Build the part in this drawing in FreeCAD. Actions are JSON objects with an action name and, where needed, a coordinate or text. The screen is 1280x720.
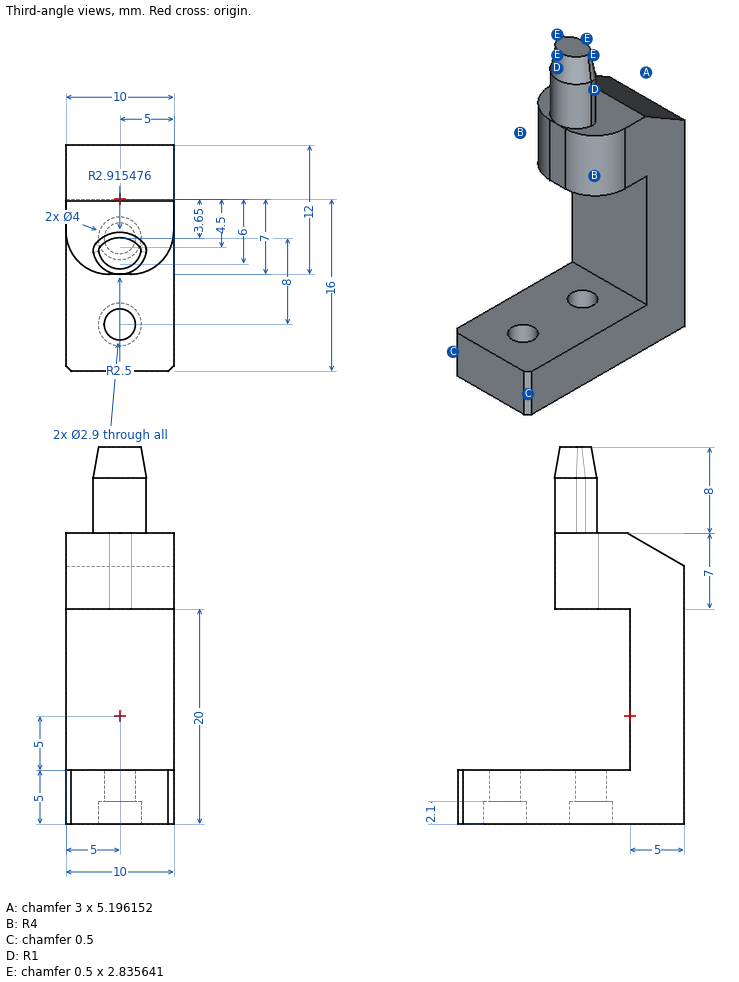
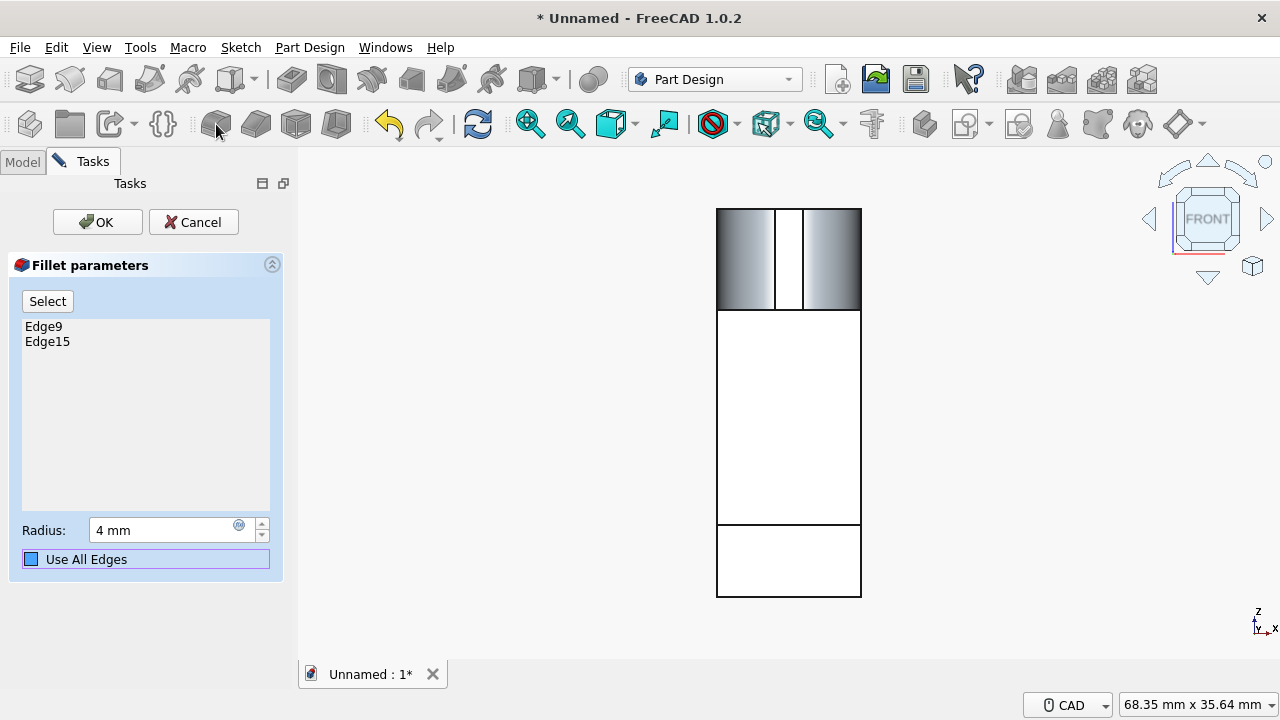
{"action": "left_click", "coordinate": [98, 222]}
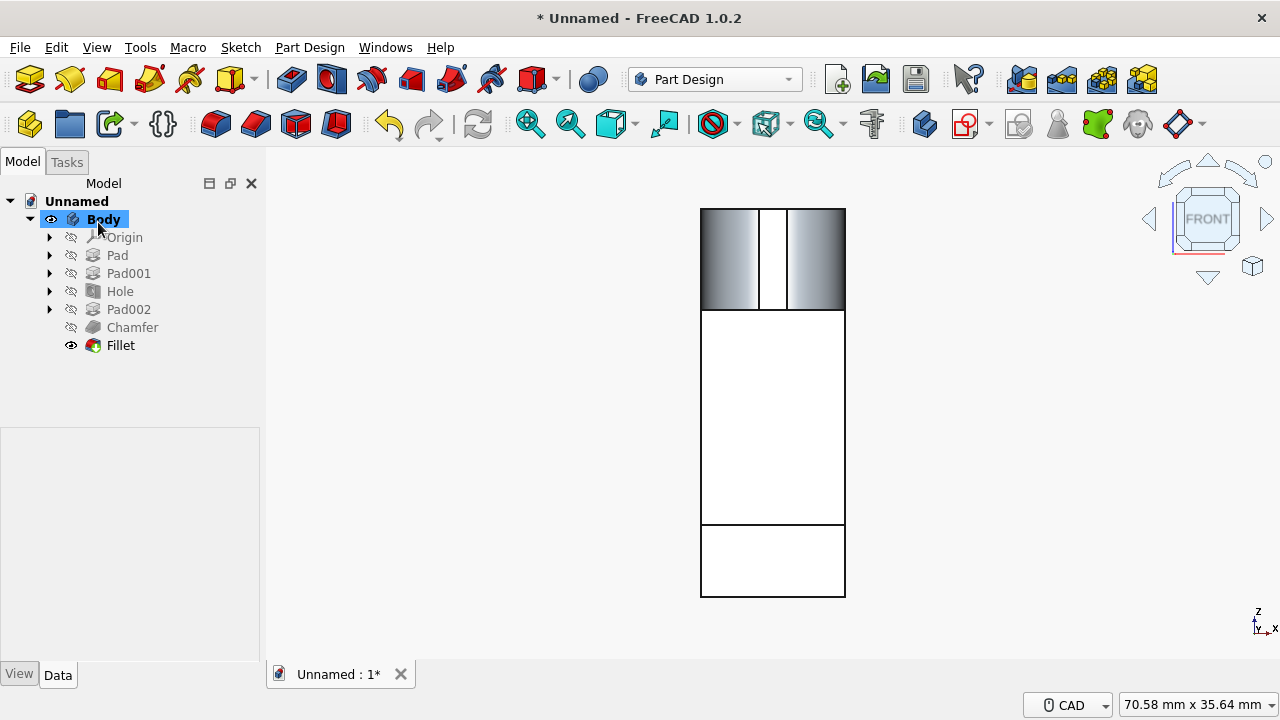
{"action": "left_click", "coordinate": [845, 560]}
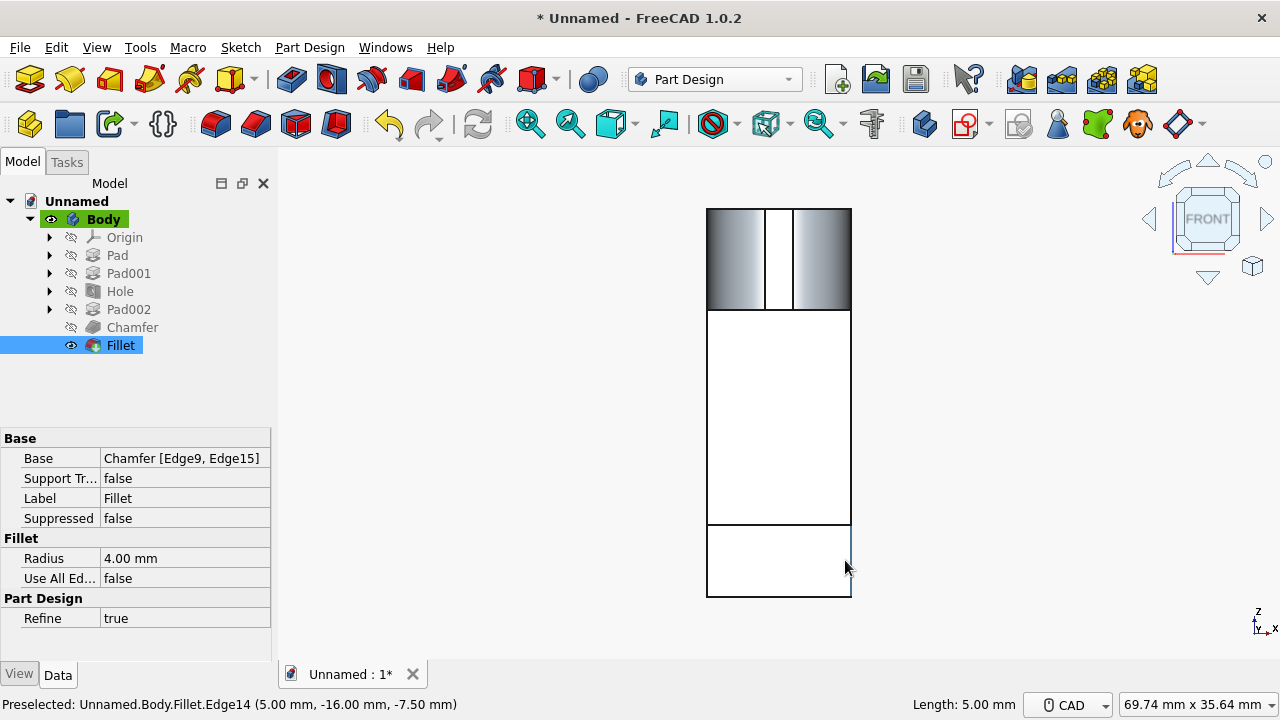
{"action": "left_click", "coordinate": [707, 560], "text": "ctrl"}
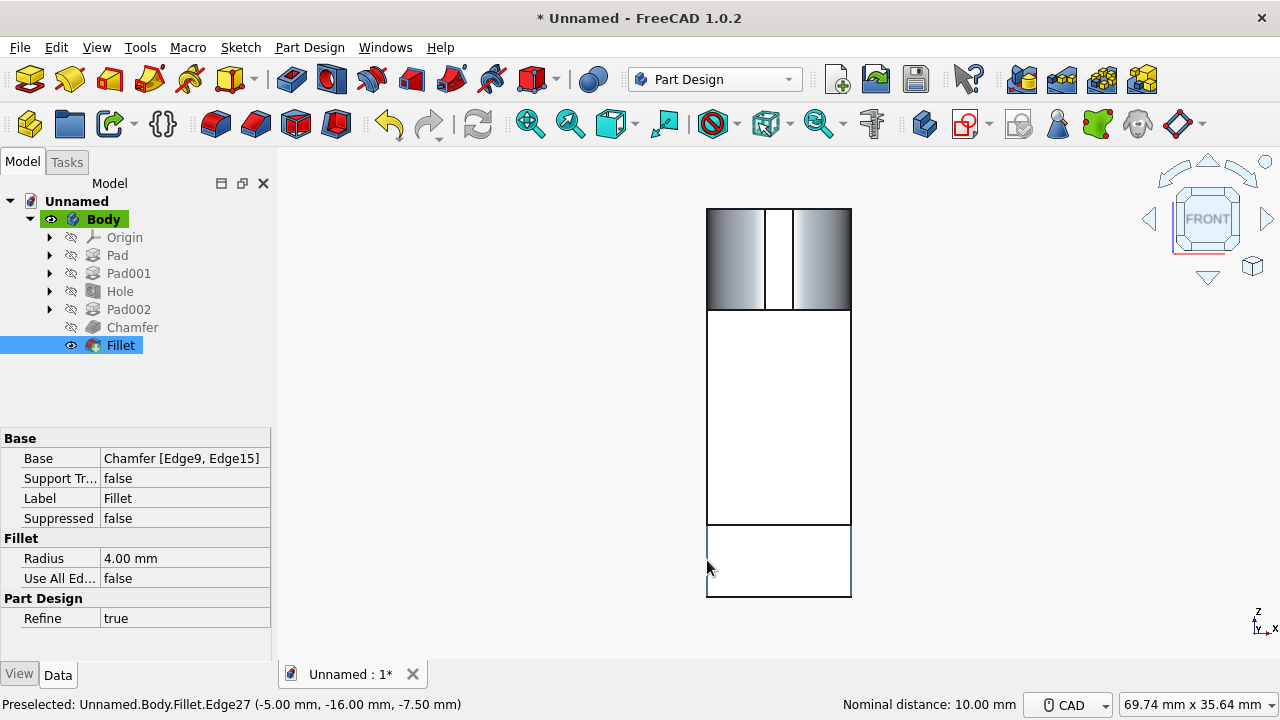
{"action": "left_click", "coordinate": [256, 124]}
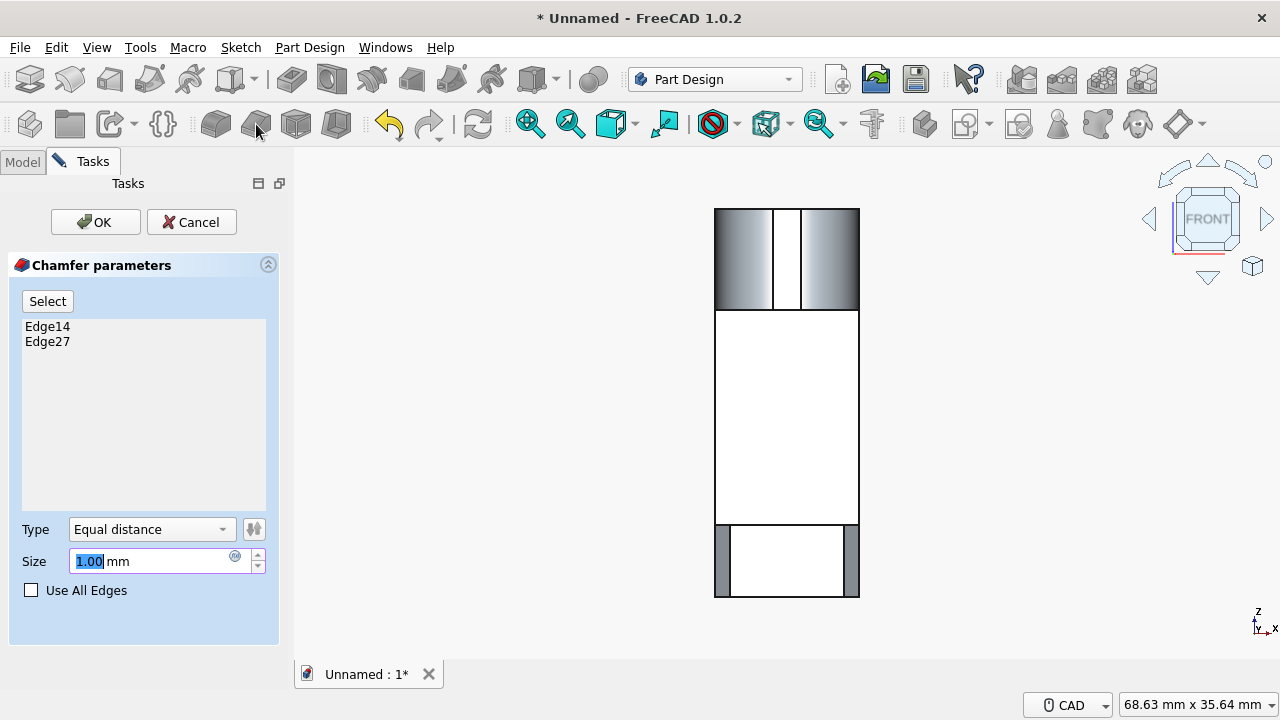
{"action": "type", "text": "0.5"}
{"action": "key", "text": "Tab"}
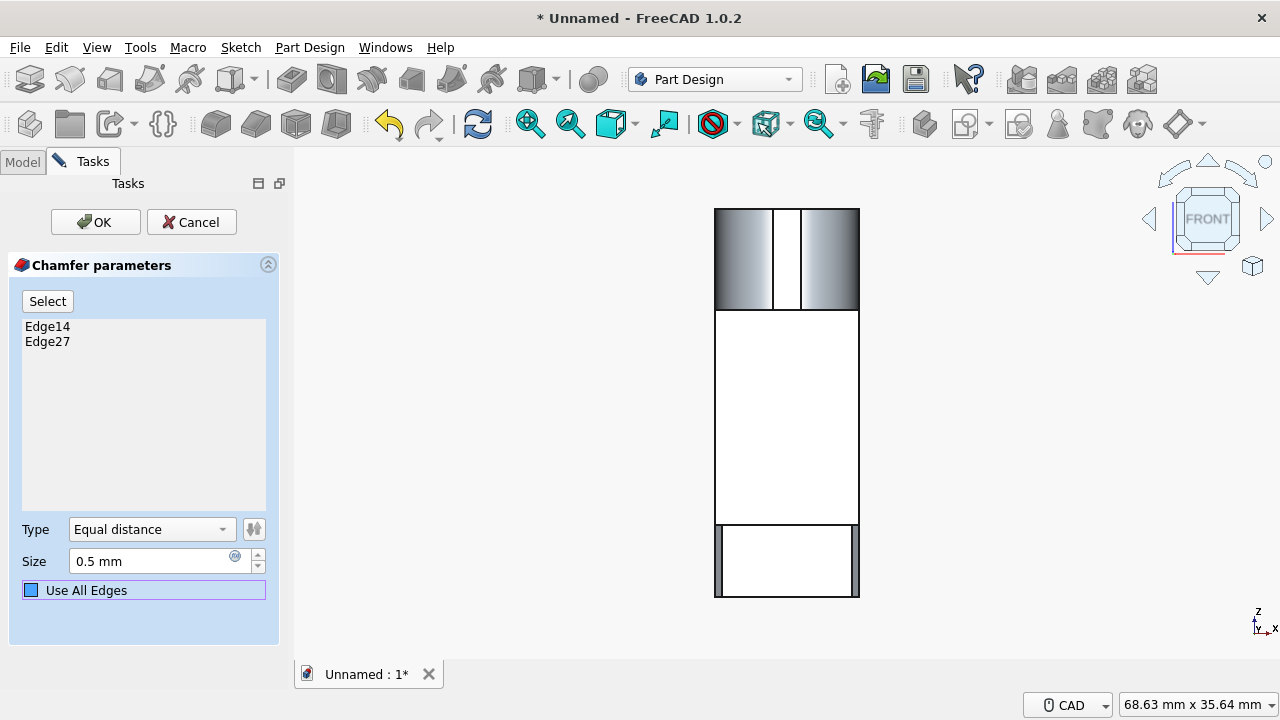
{"action": "left_click", "coordinate": [96, 222]}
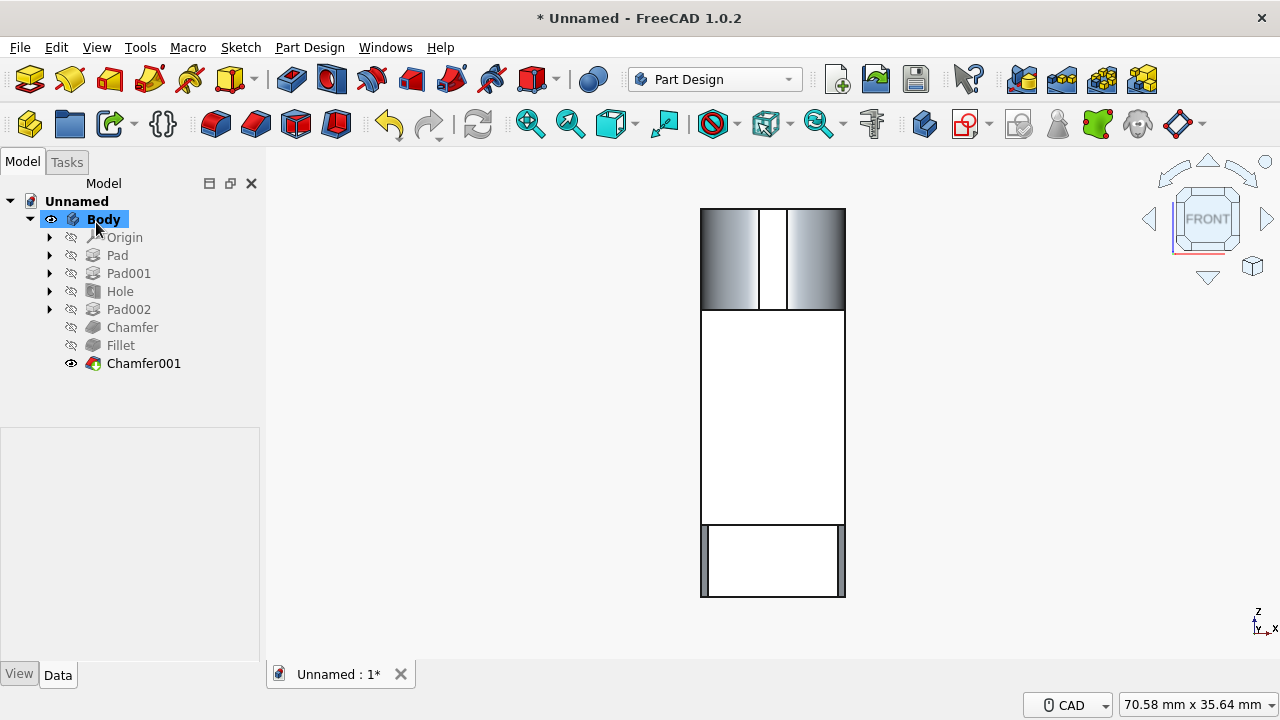
{"action": "key", "text": "0"}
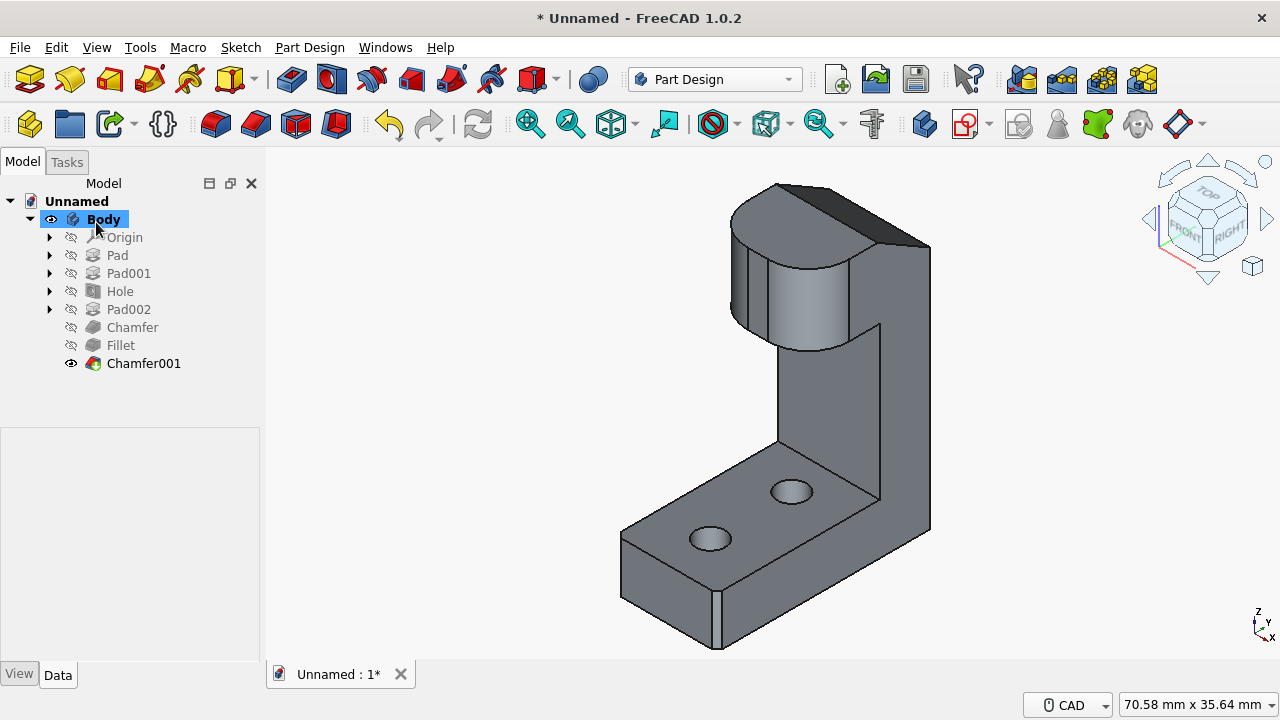
{"action": "left_click", "coordinate": [792, 232]}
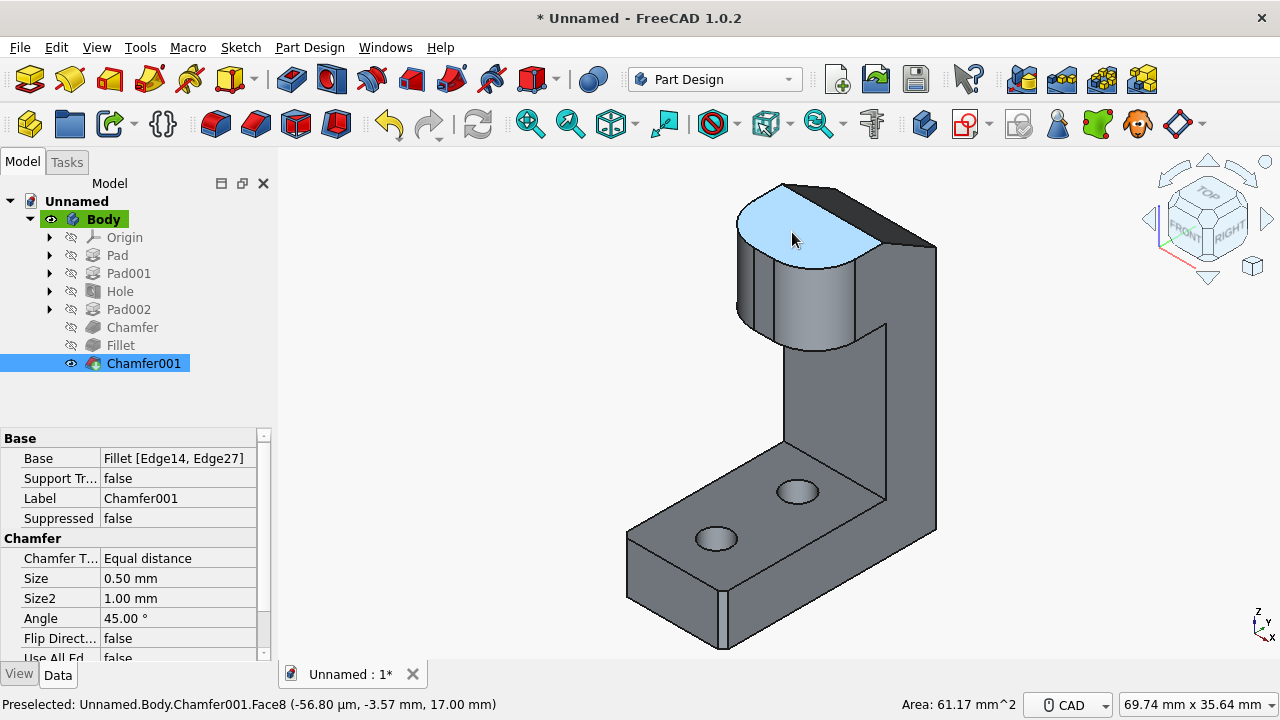
{"action": "left_click", "coordinate": [966, 124]}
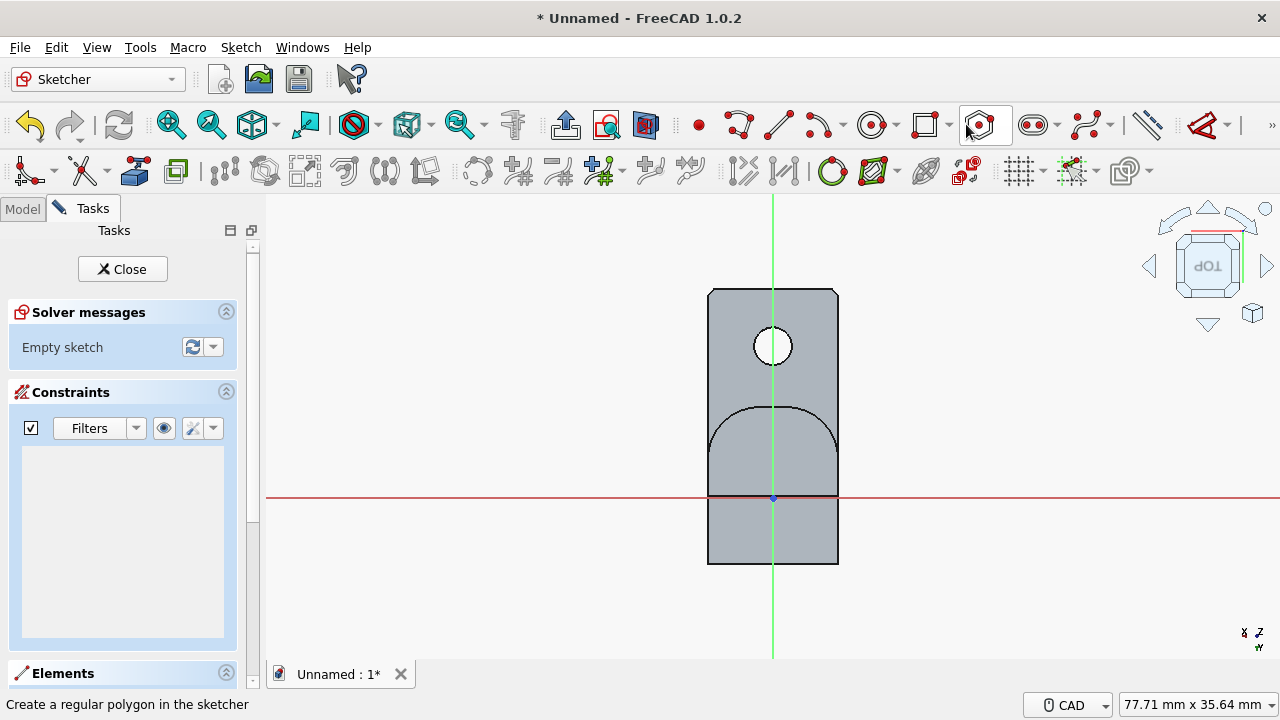
{"action": "scroll", "coordinate": [803, 464], "scroll_direction": "up", "scroll_amount": 6}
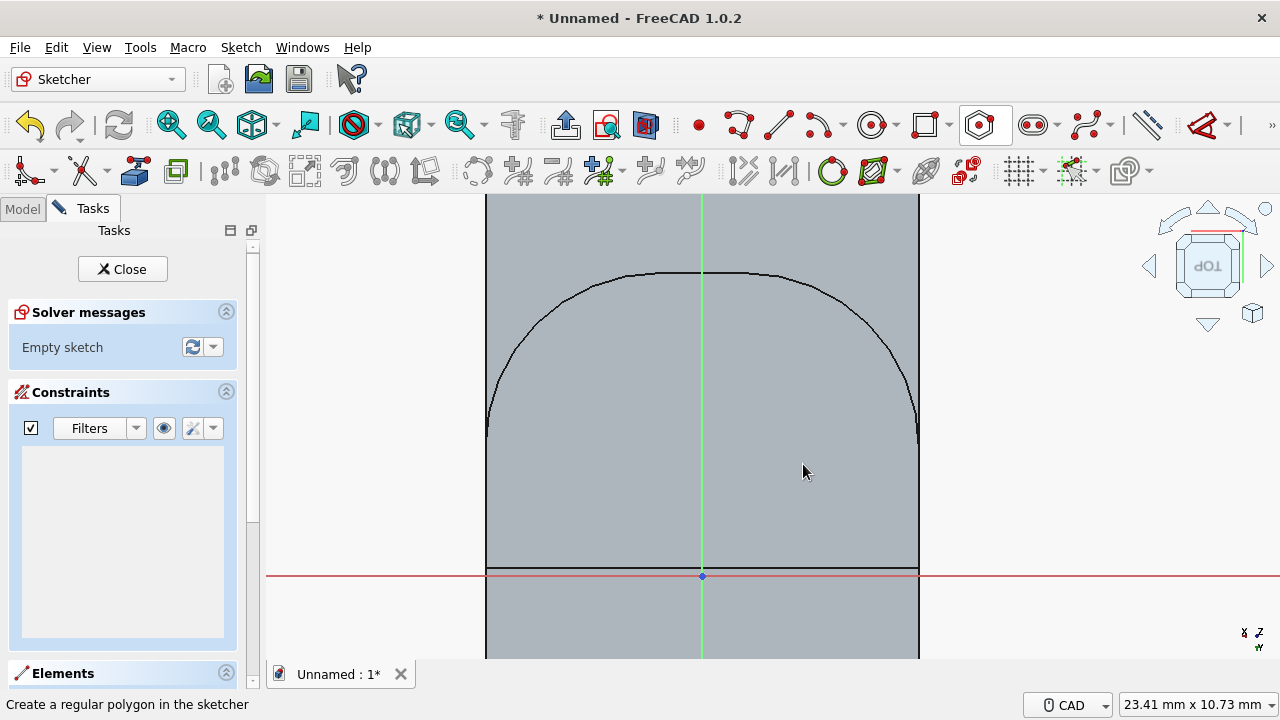
{"action": "key", "text": "g 3 a"}